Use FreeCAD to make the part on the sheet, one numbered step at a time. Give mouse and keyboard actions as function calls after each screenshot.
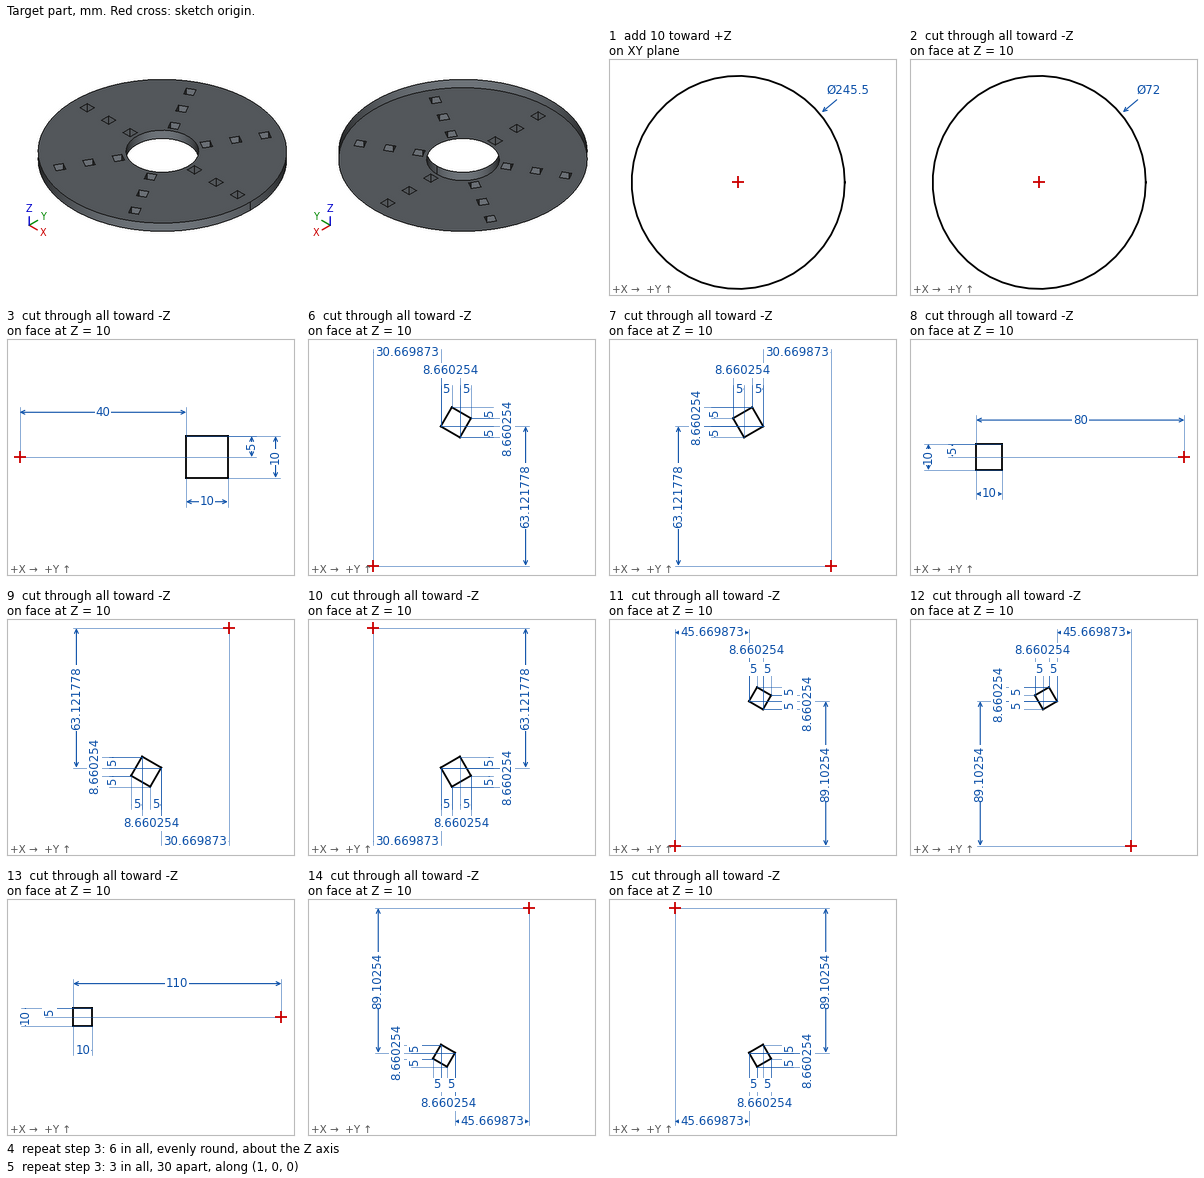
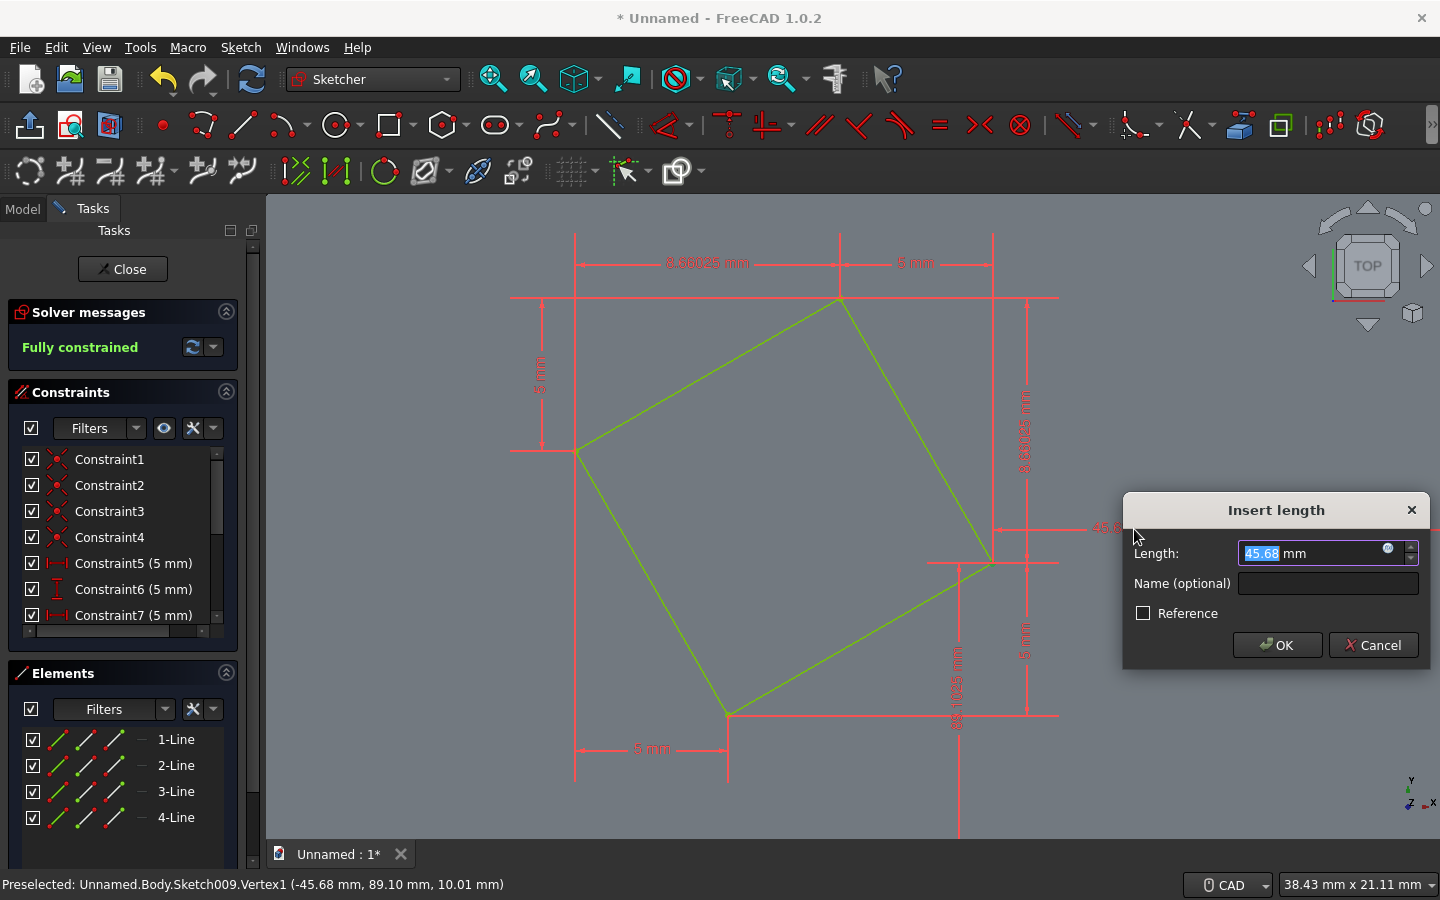
text(45.669873)
key(Return)
key(Escape)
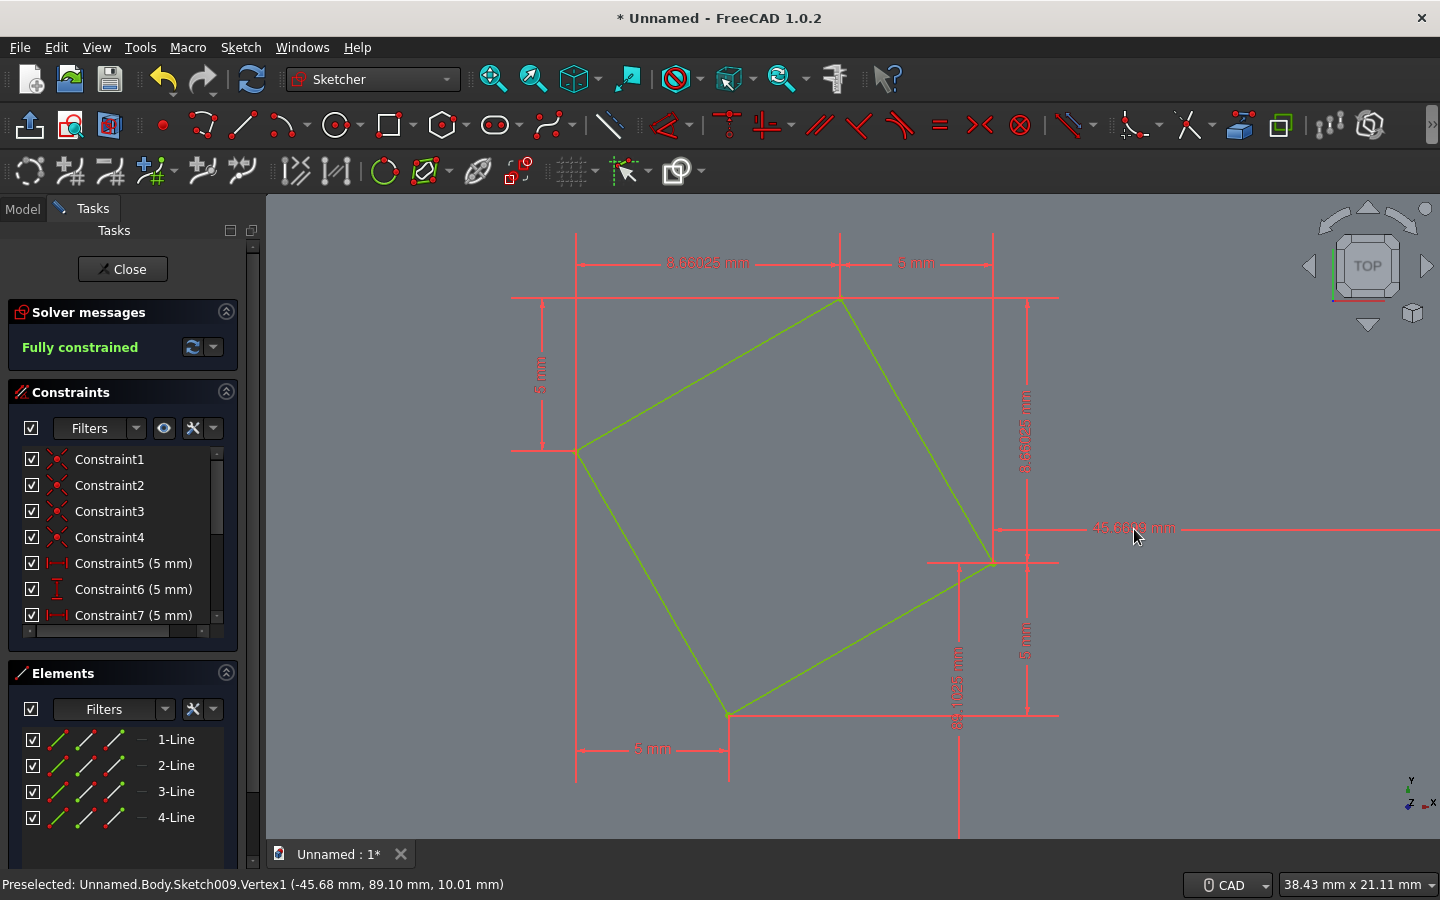
click(123, 269)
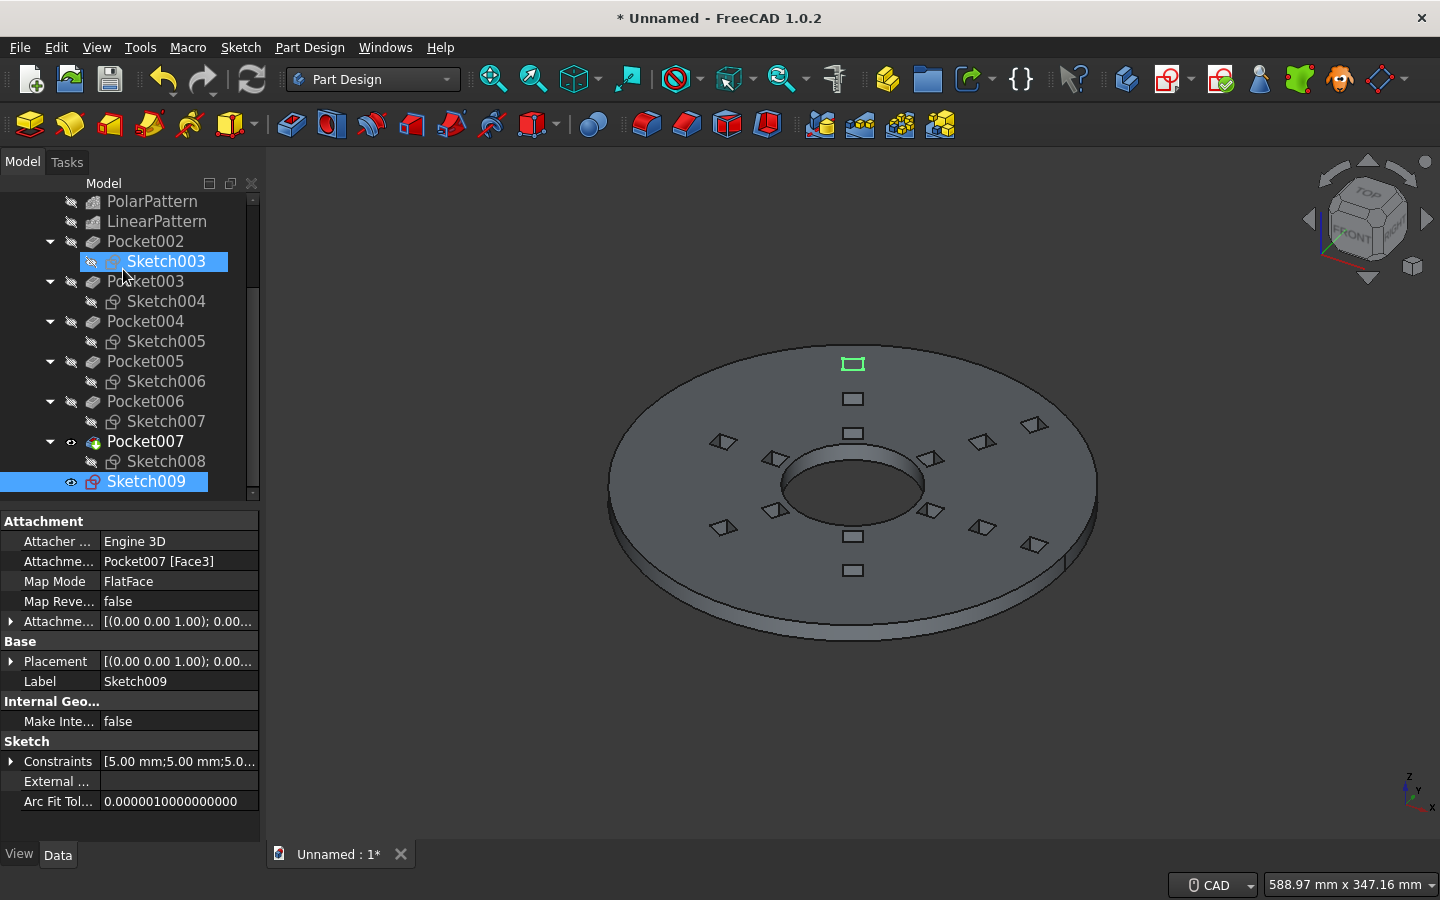
click(292, 124)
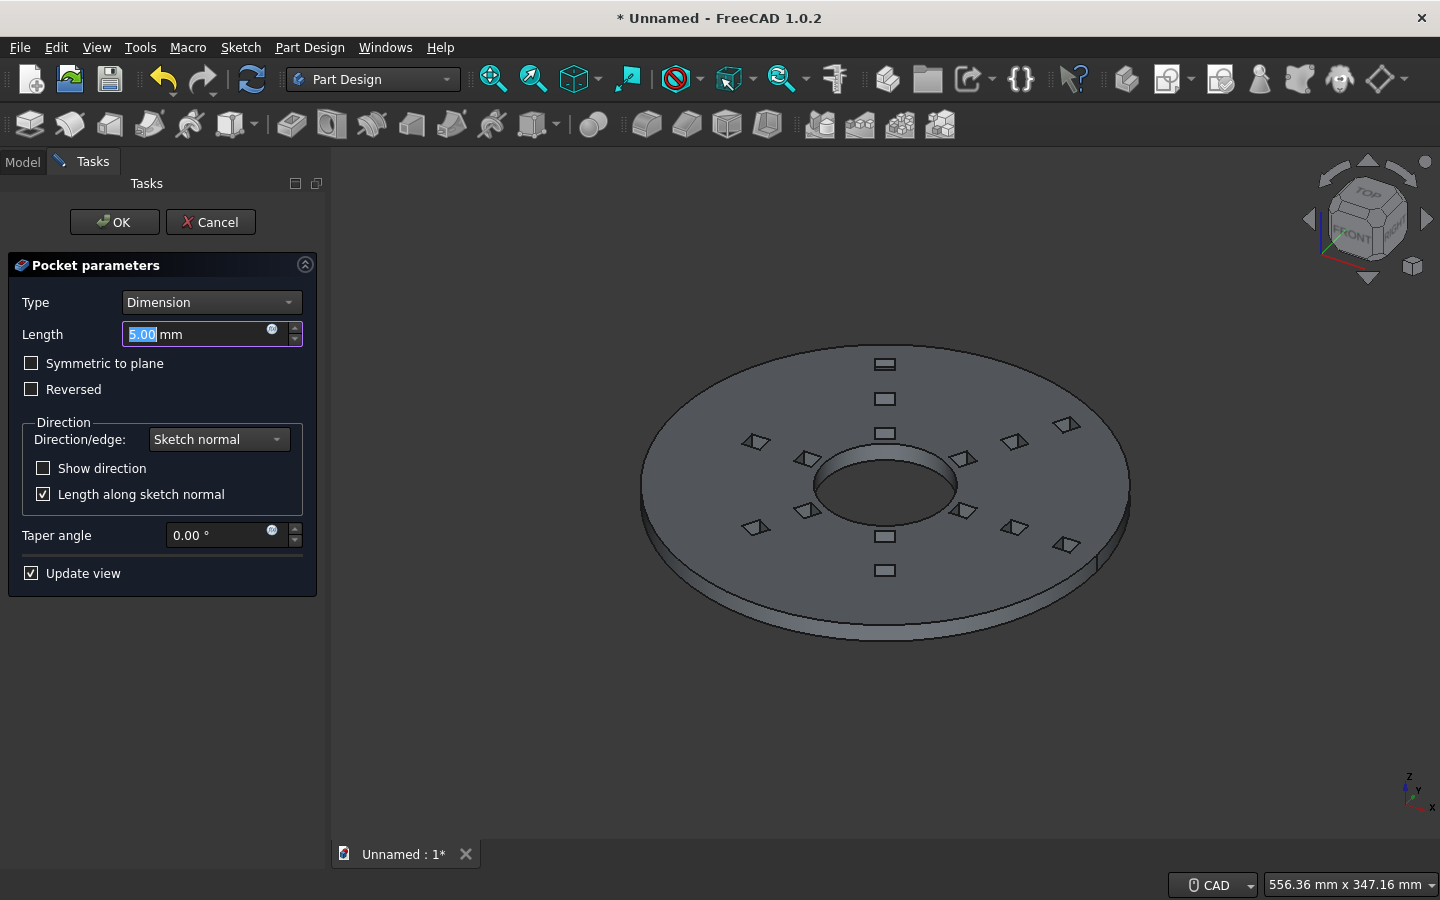
click(212, 302)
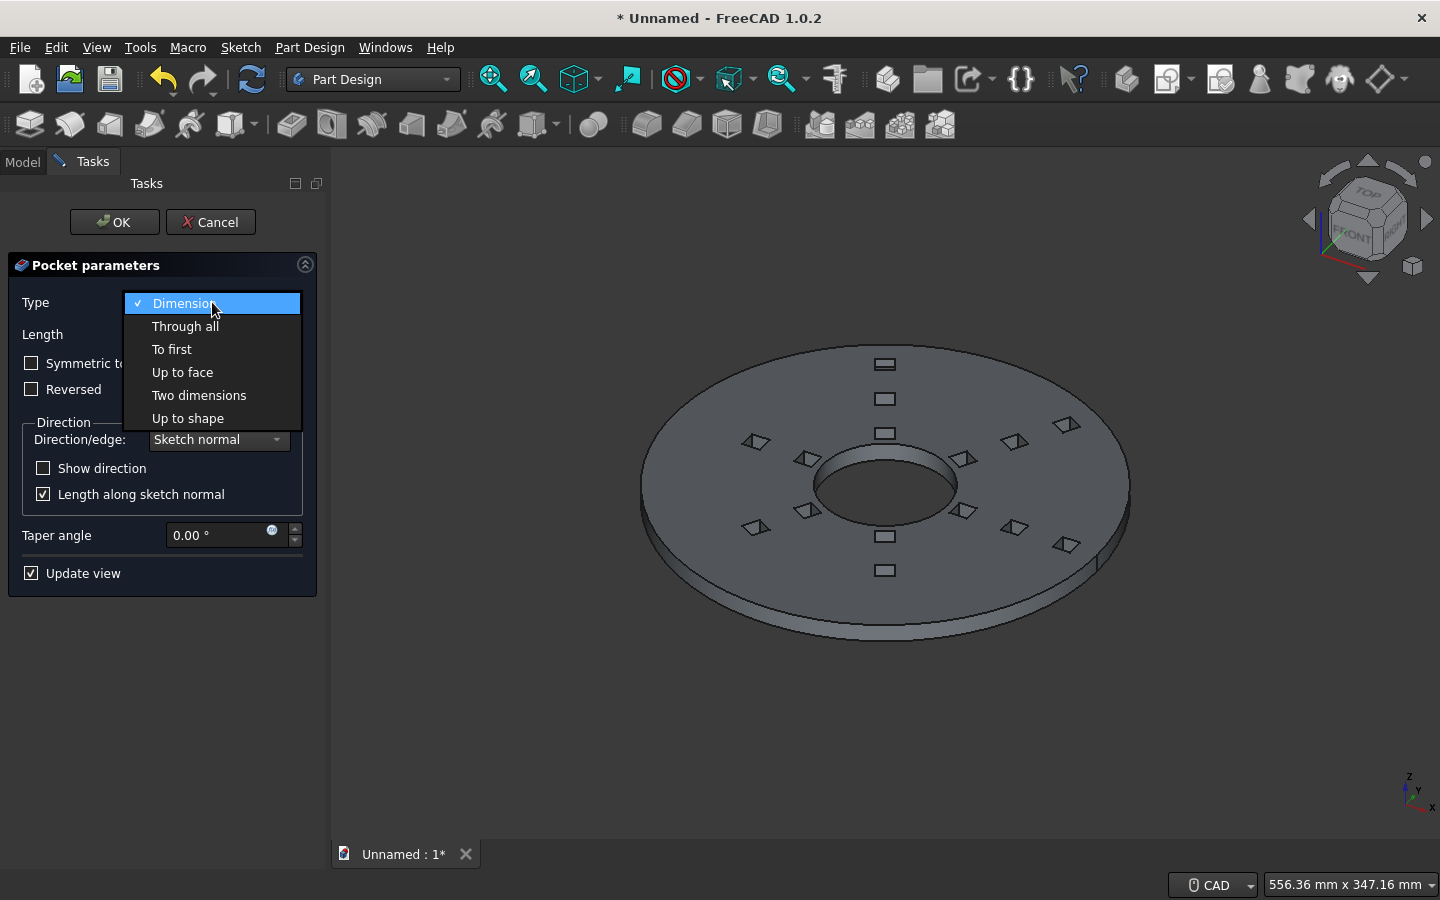
click(212, 326)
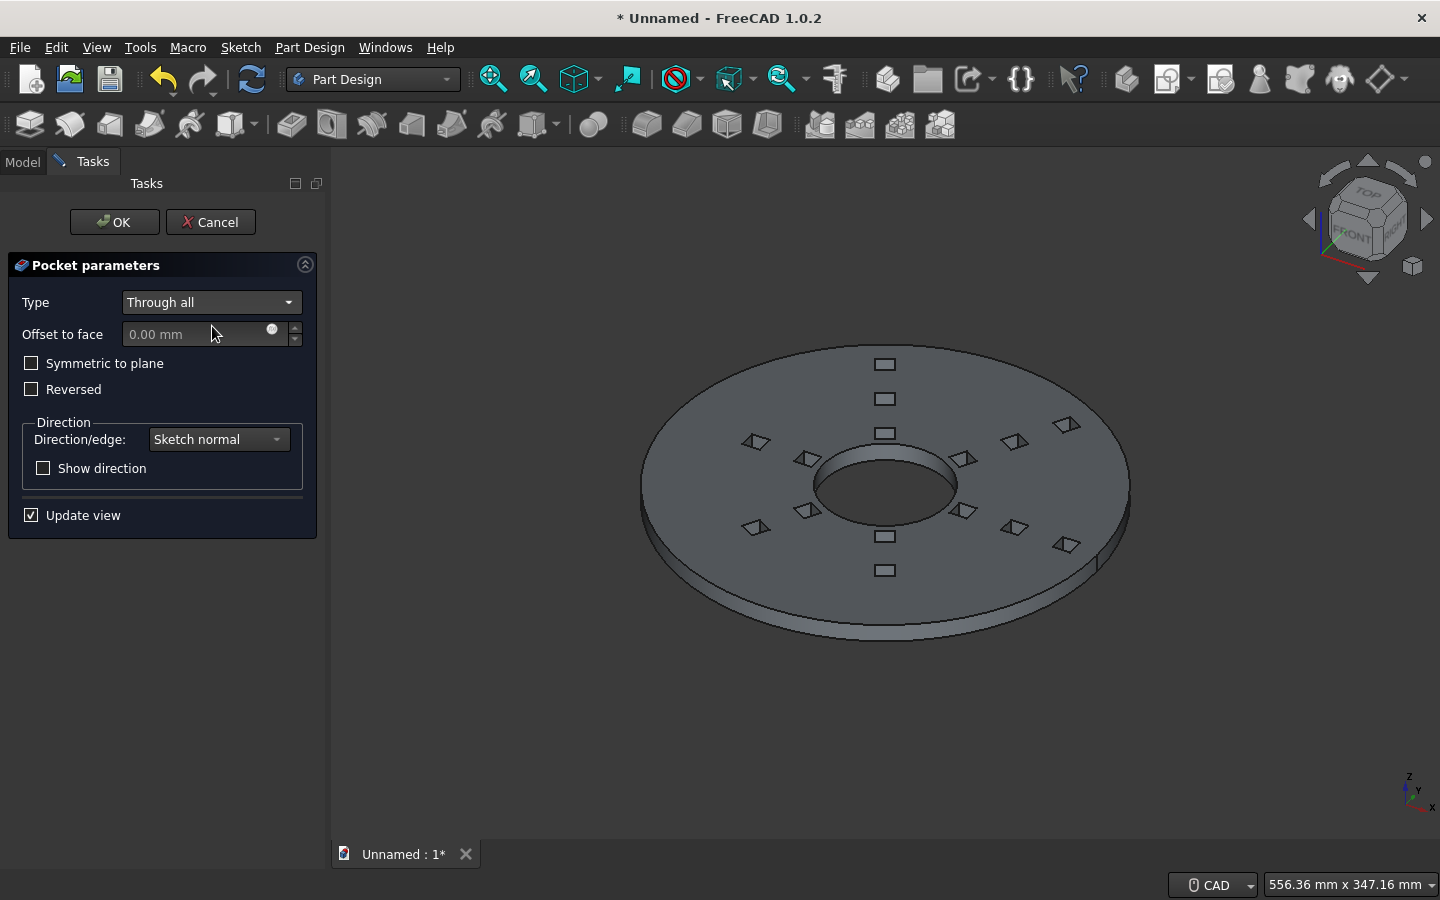
click(115, 222)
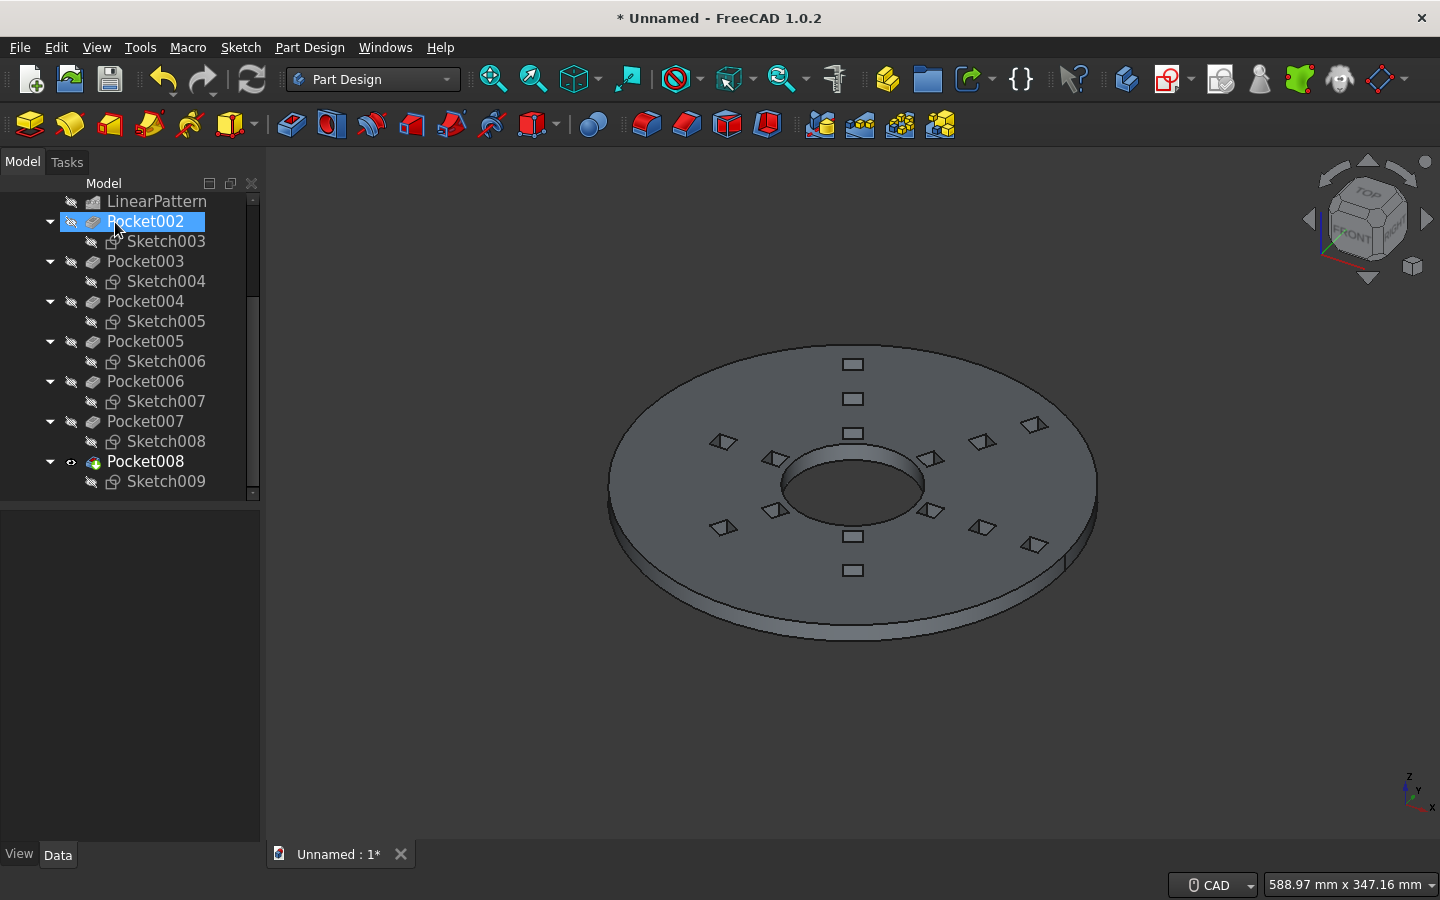
click(923, 414)